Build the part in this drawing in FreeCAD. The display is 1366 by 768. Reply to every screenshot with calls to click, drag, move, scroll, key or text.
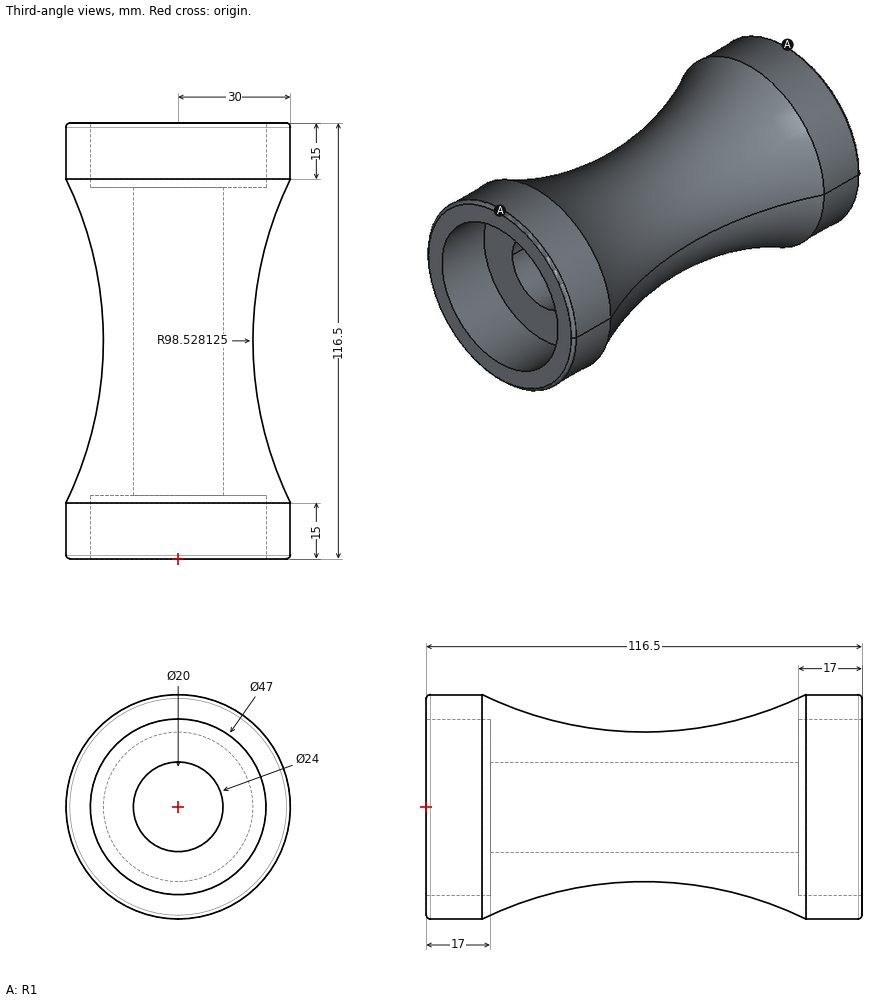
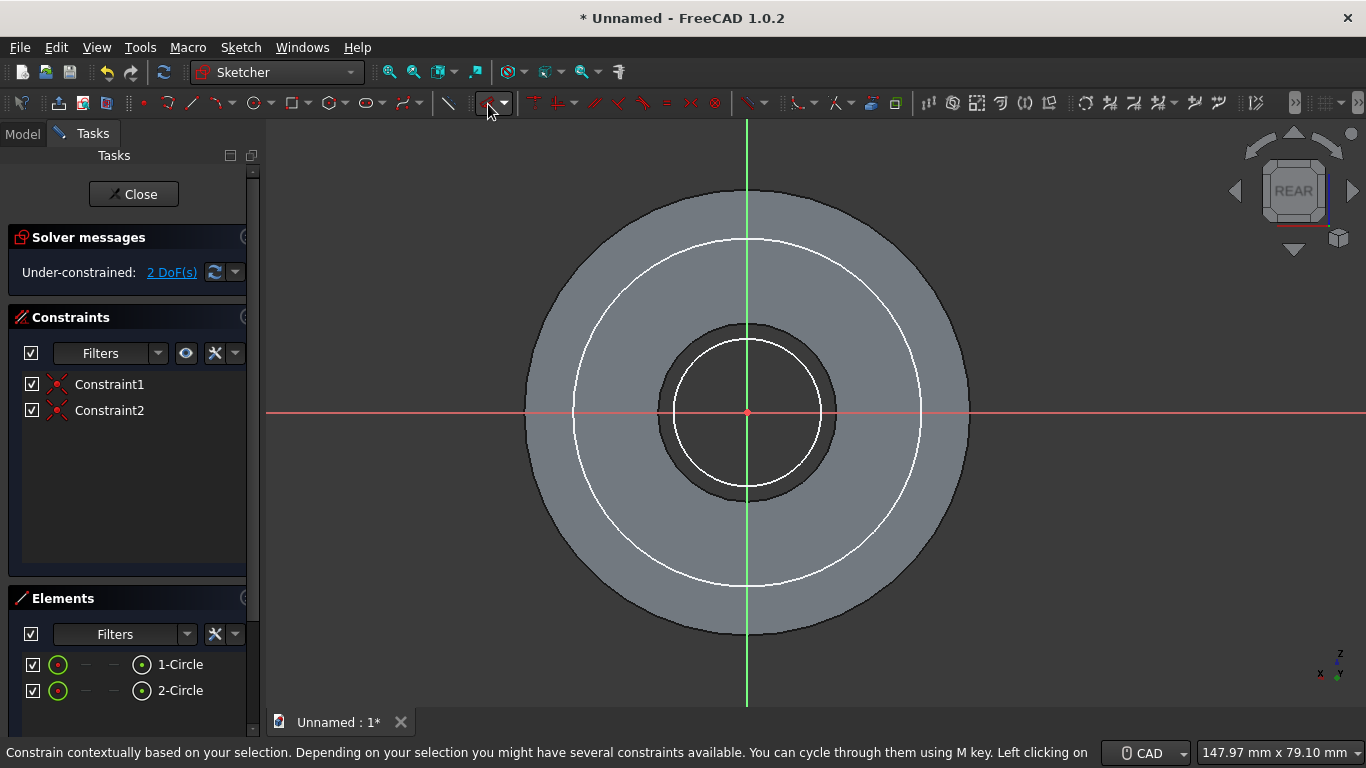
click(870, 289)
click(893, 266)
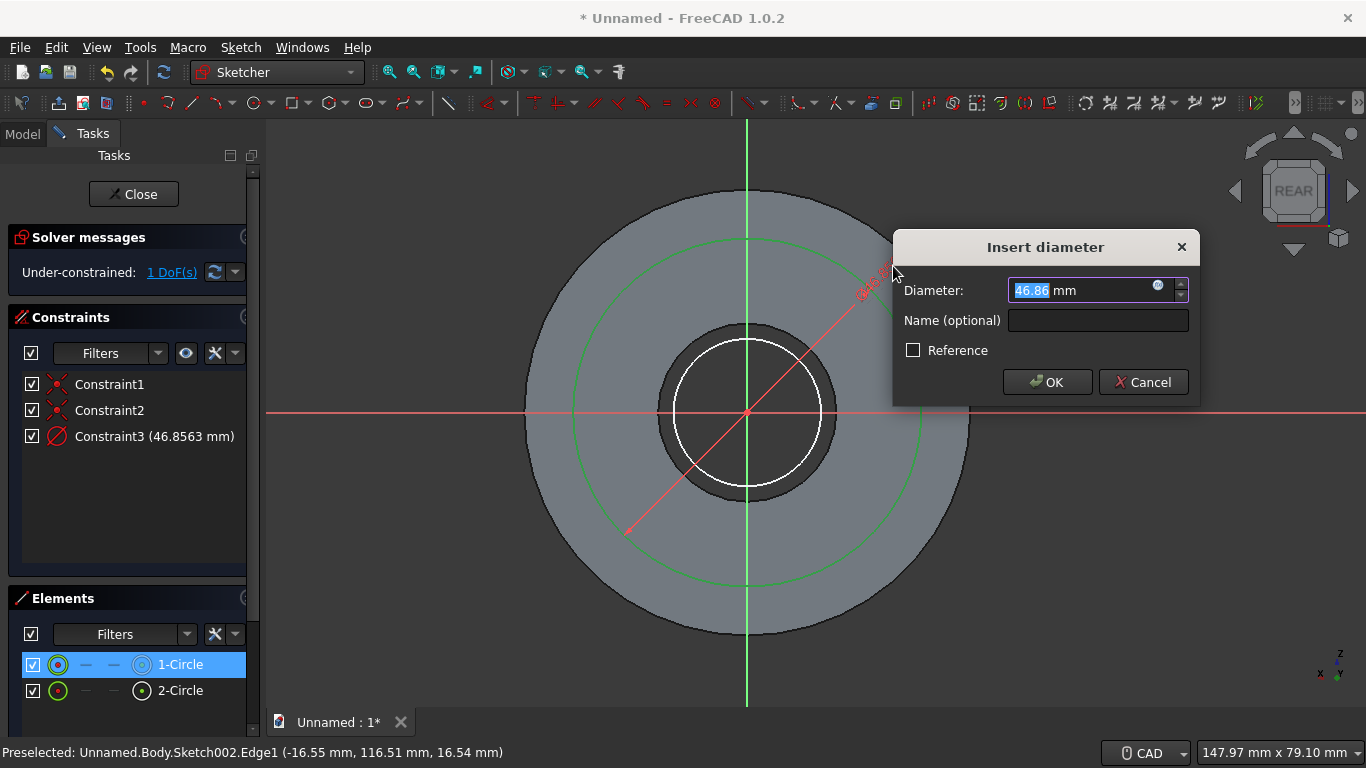
text(47)
key(Return)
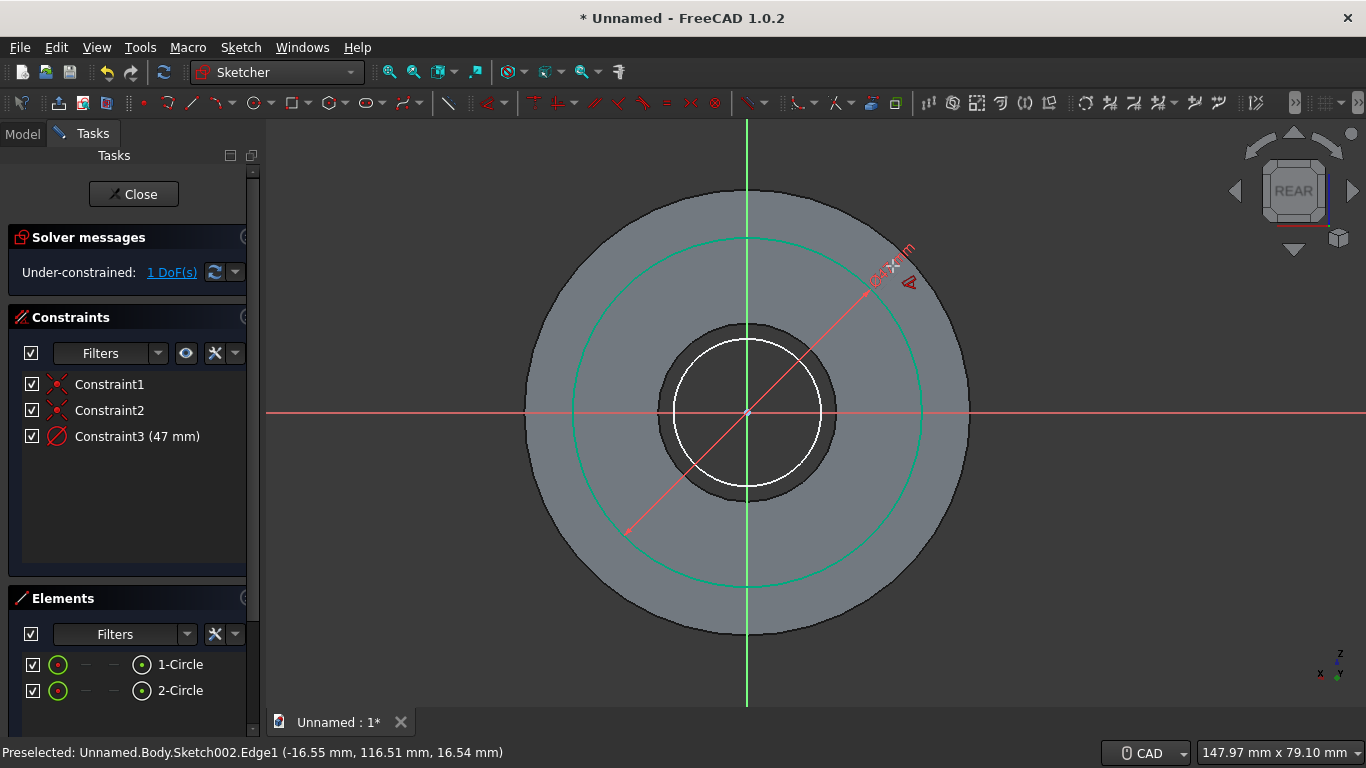
click(799, 360)
click(821, 337)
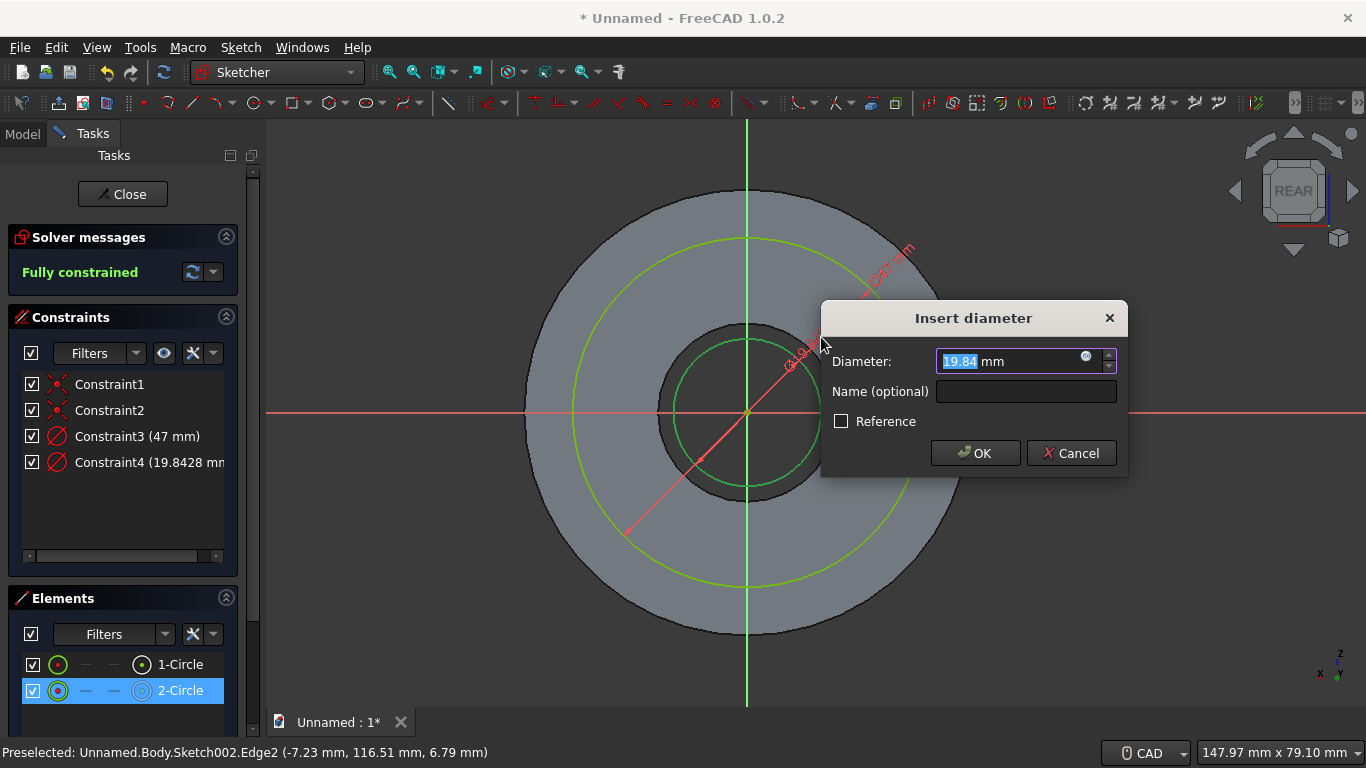
text(20)
key(Return)
key(Escape)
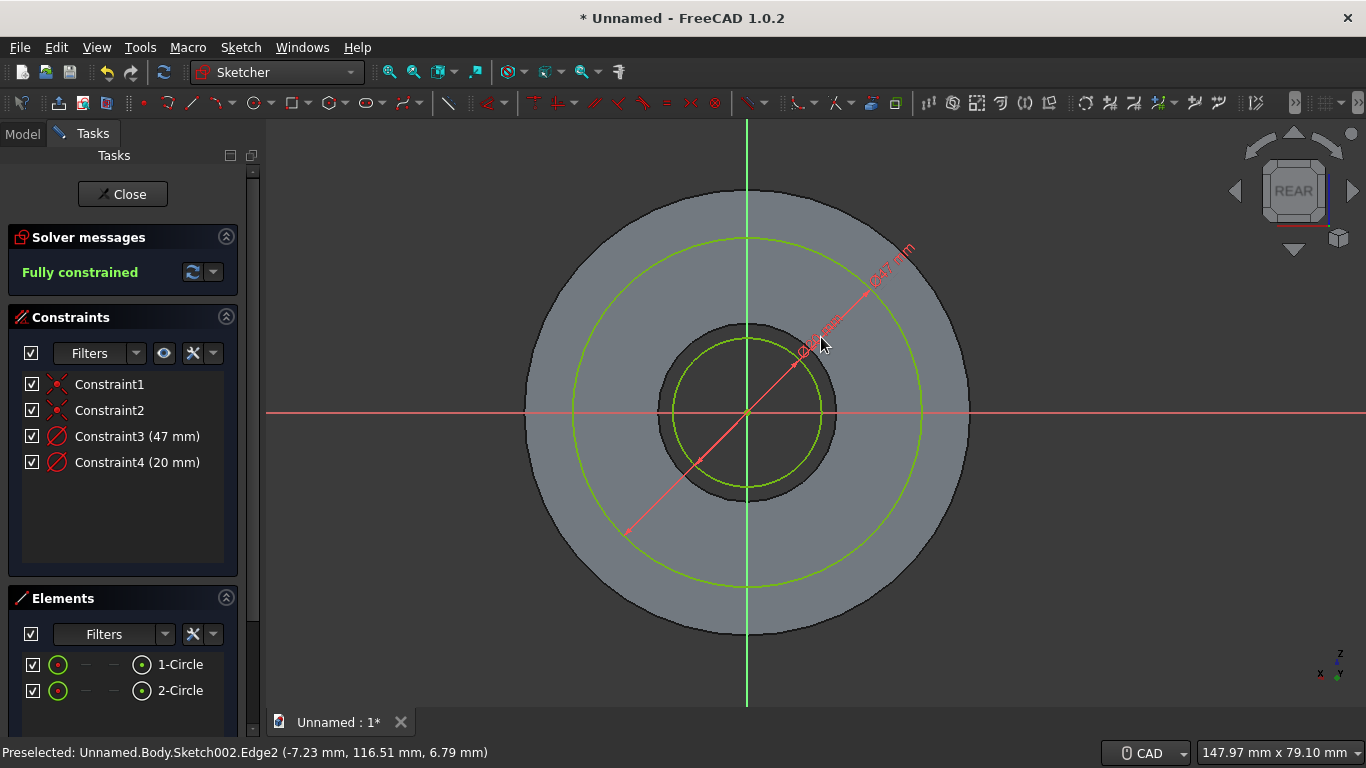
click(123, 194)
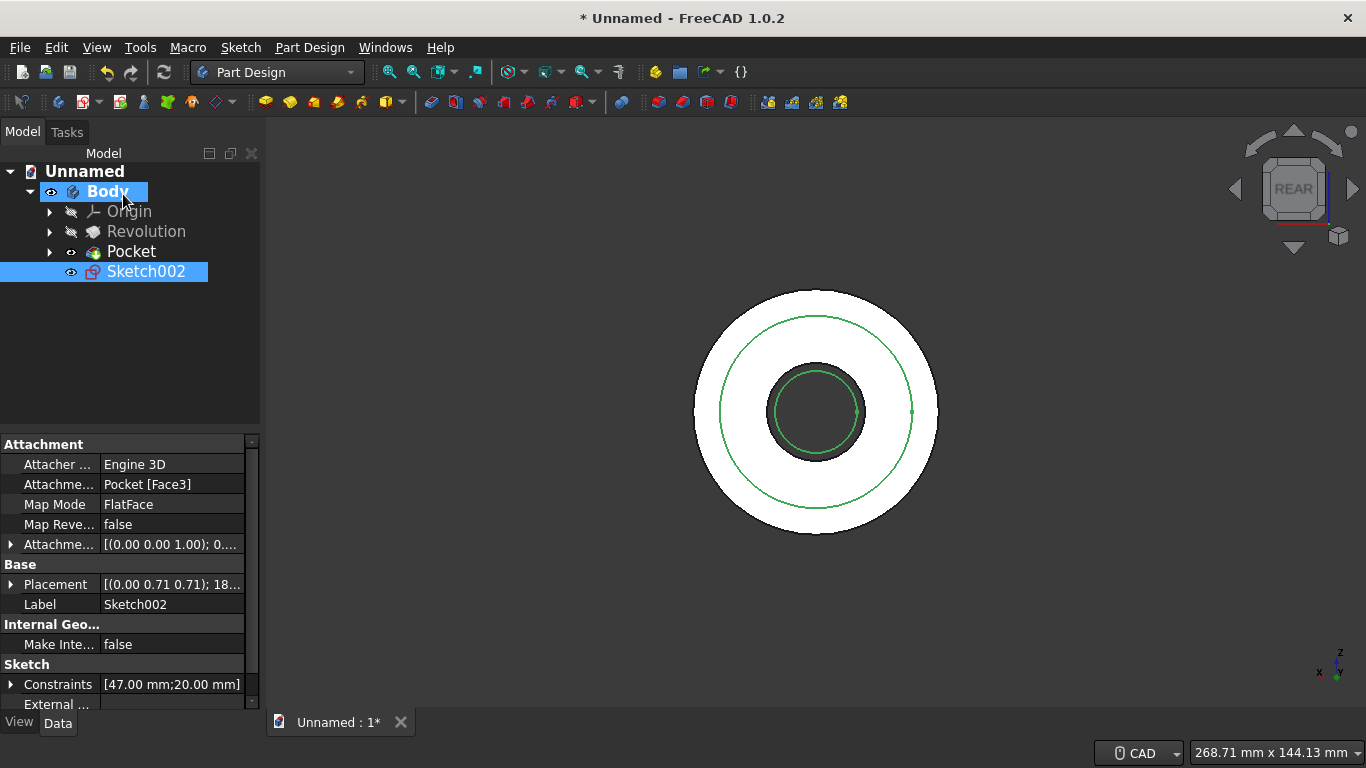
click(432, 102)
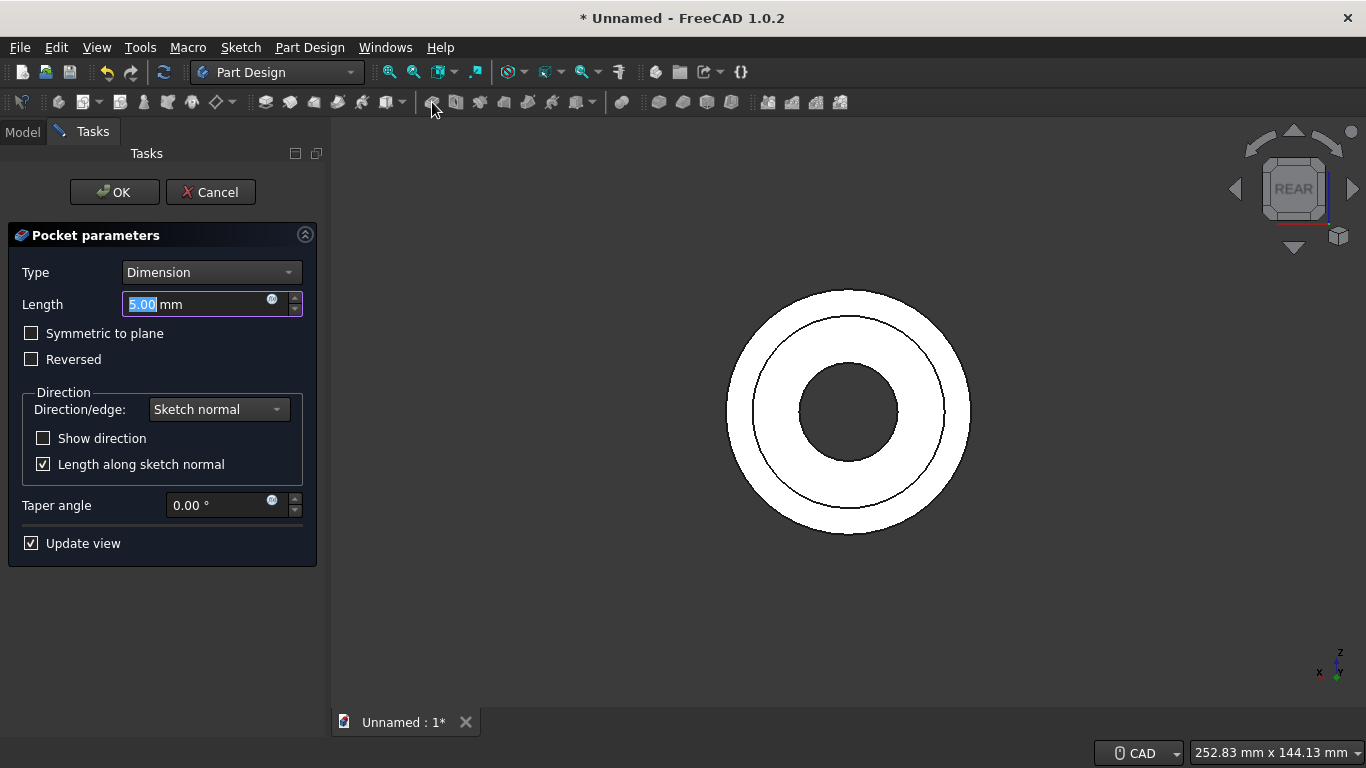
text(17)
key(Tab)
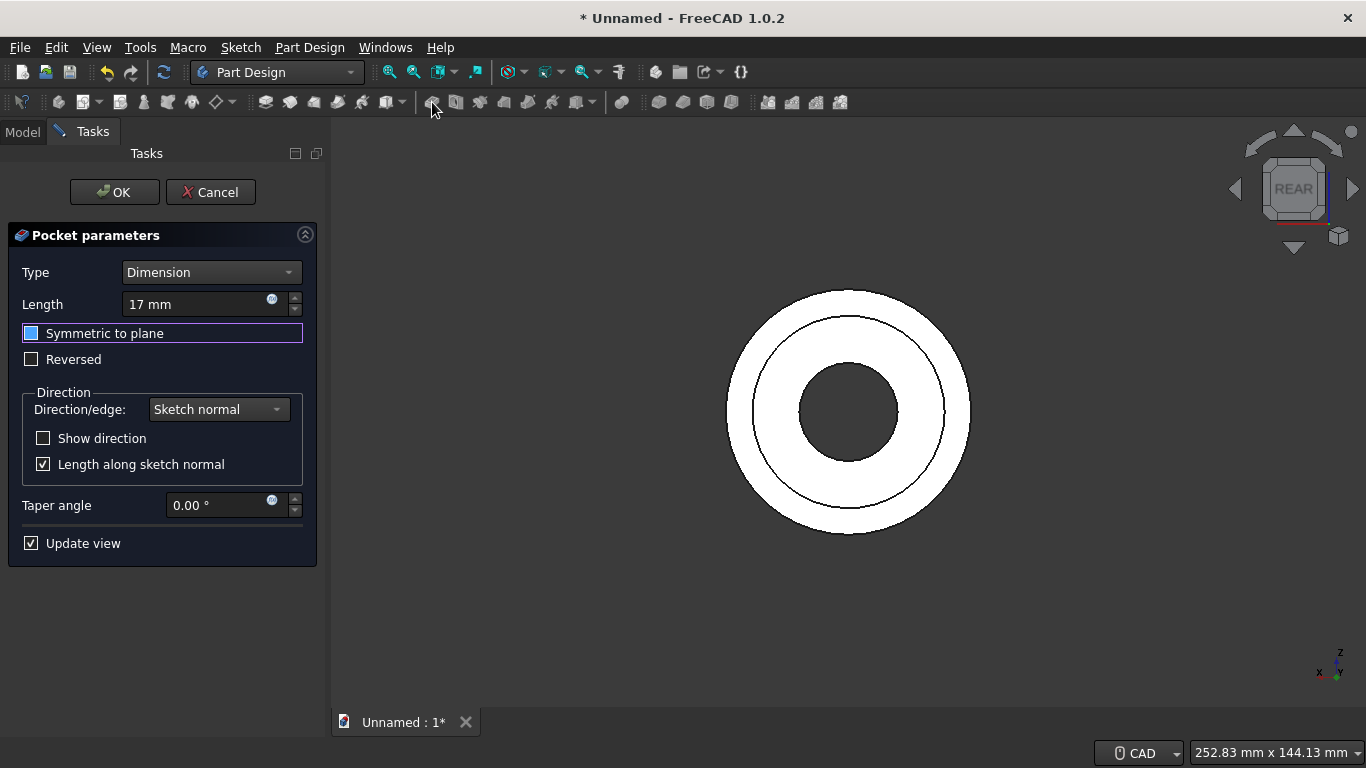
click(115, 192)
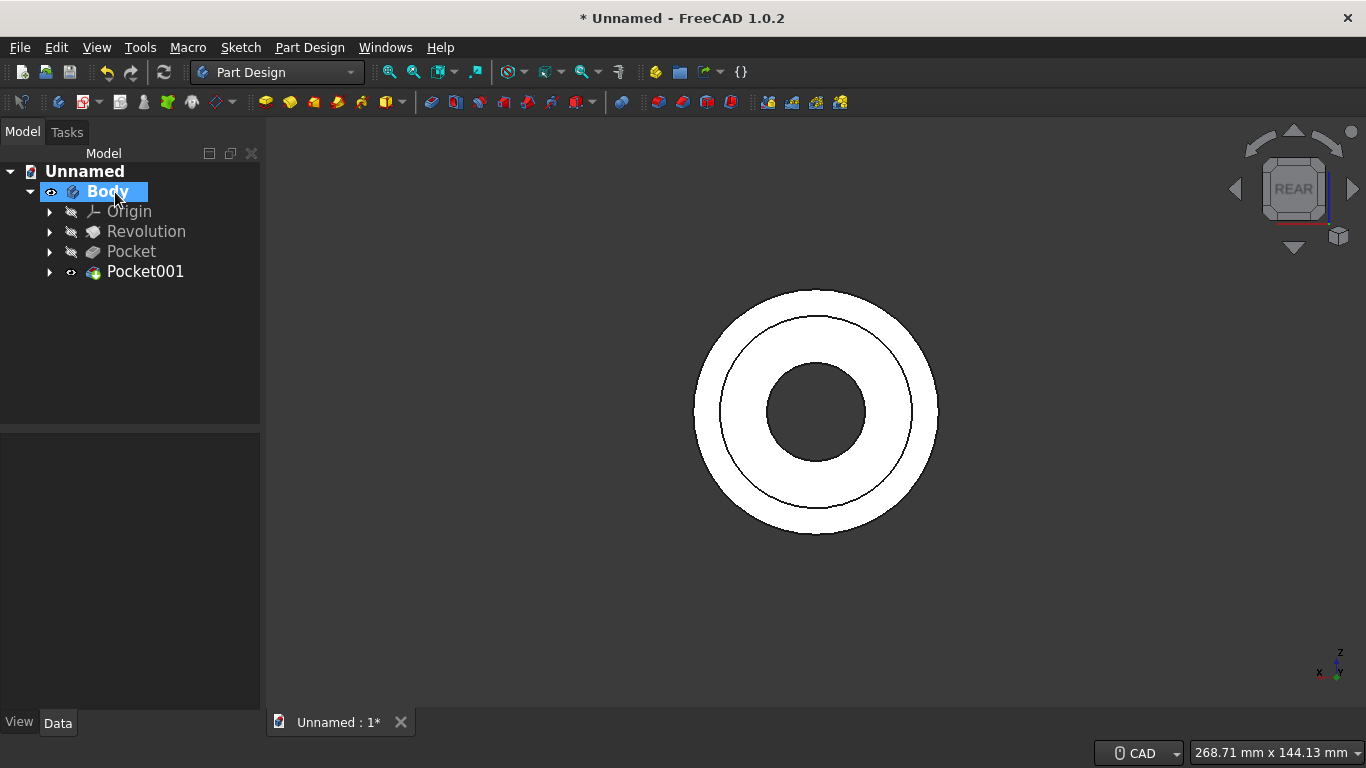
click(390, 72)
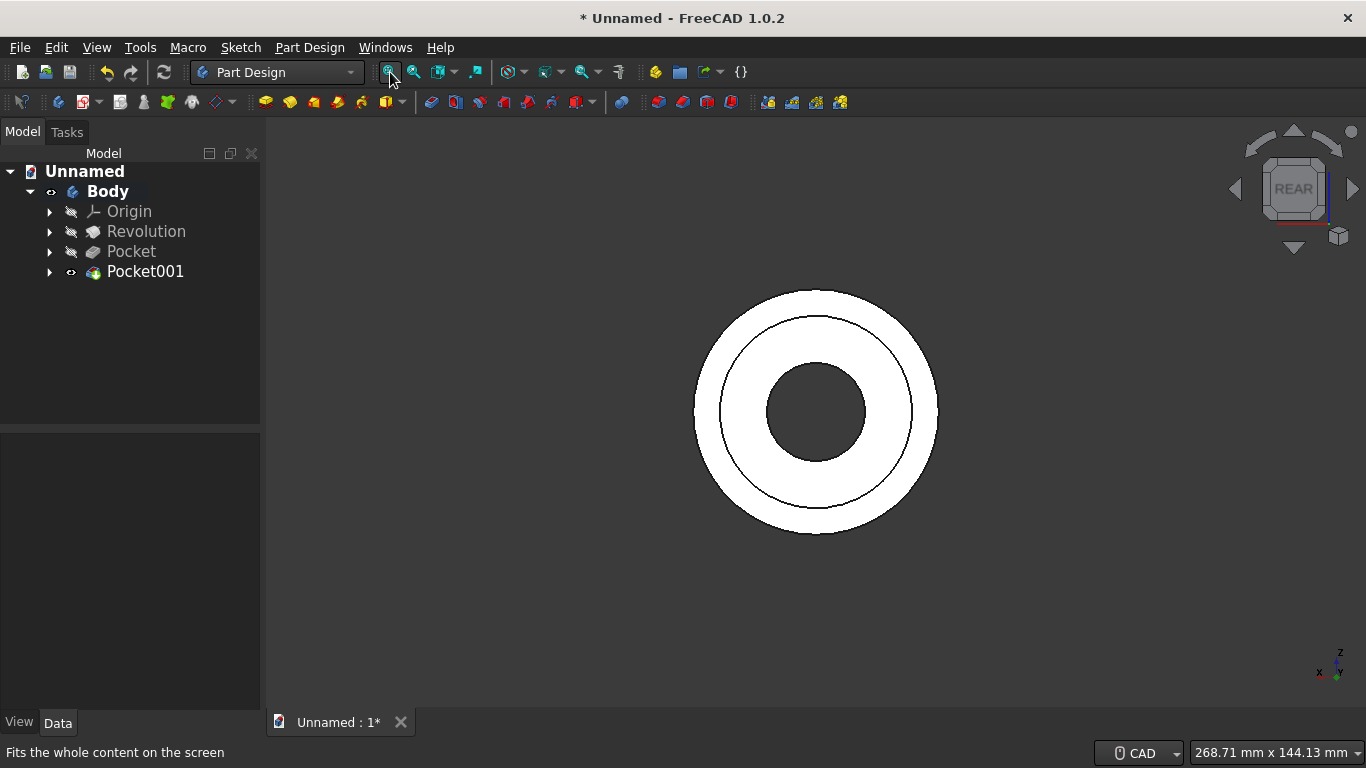
click(50, 212)